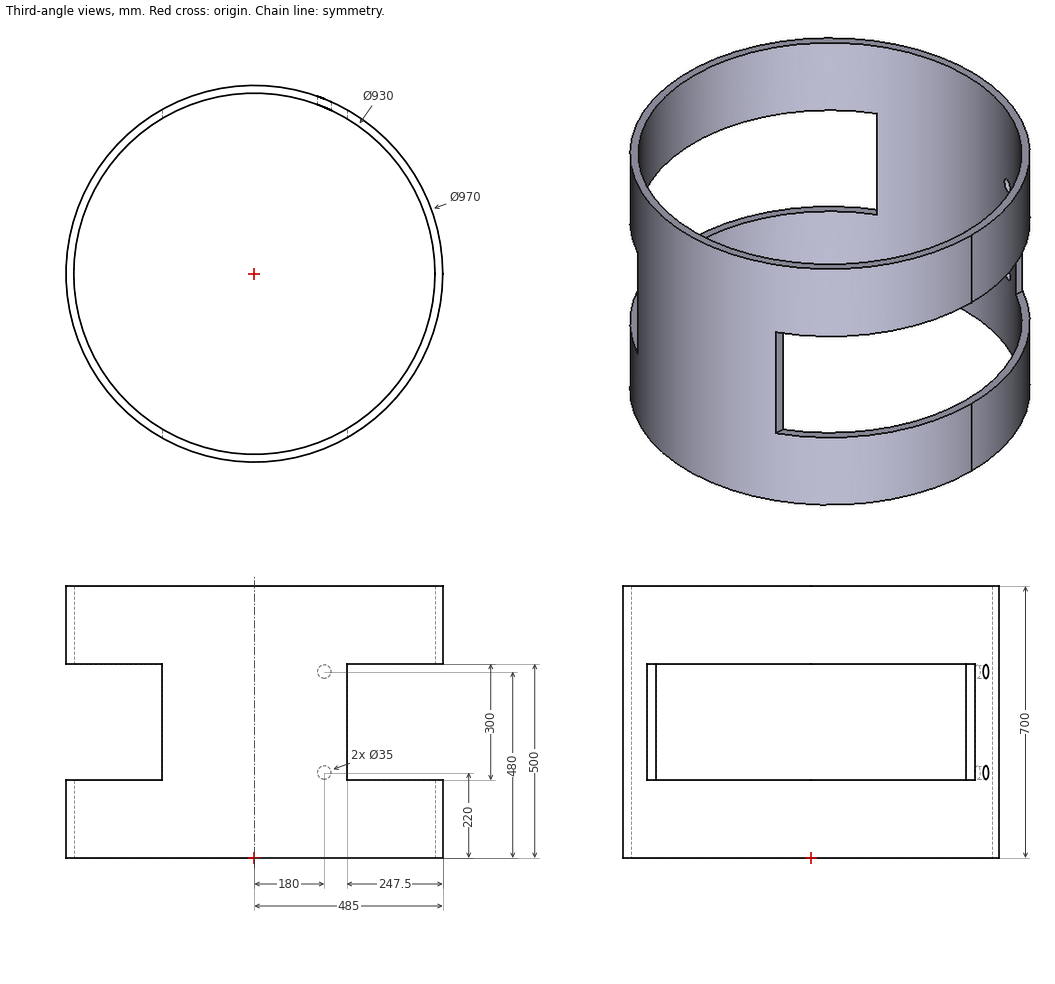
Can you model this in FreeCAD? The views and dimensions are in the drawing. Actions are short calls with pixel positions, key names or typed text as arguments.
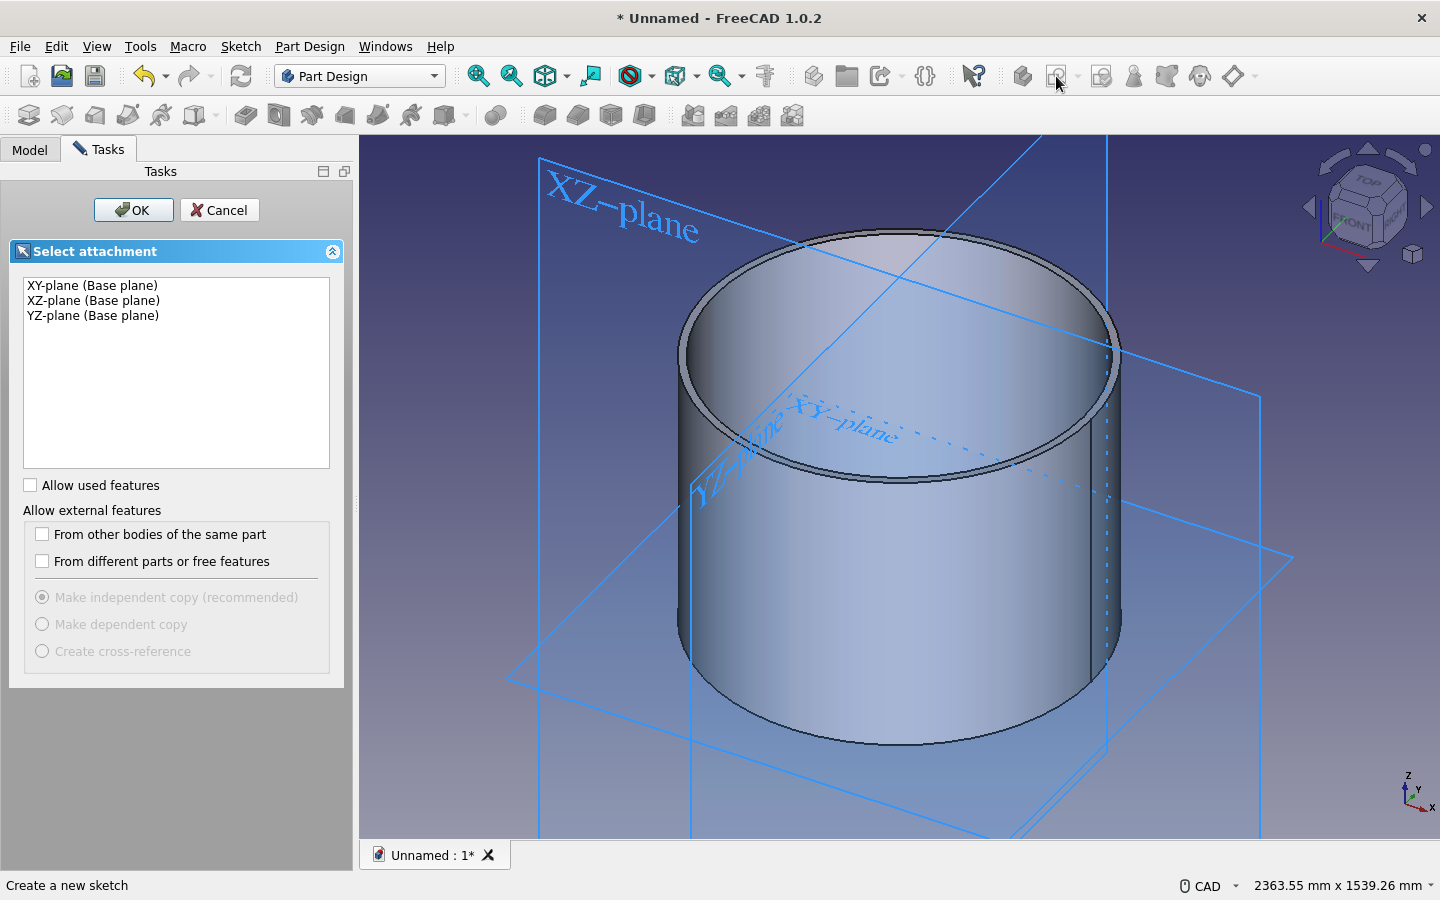
click(84, 300)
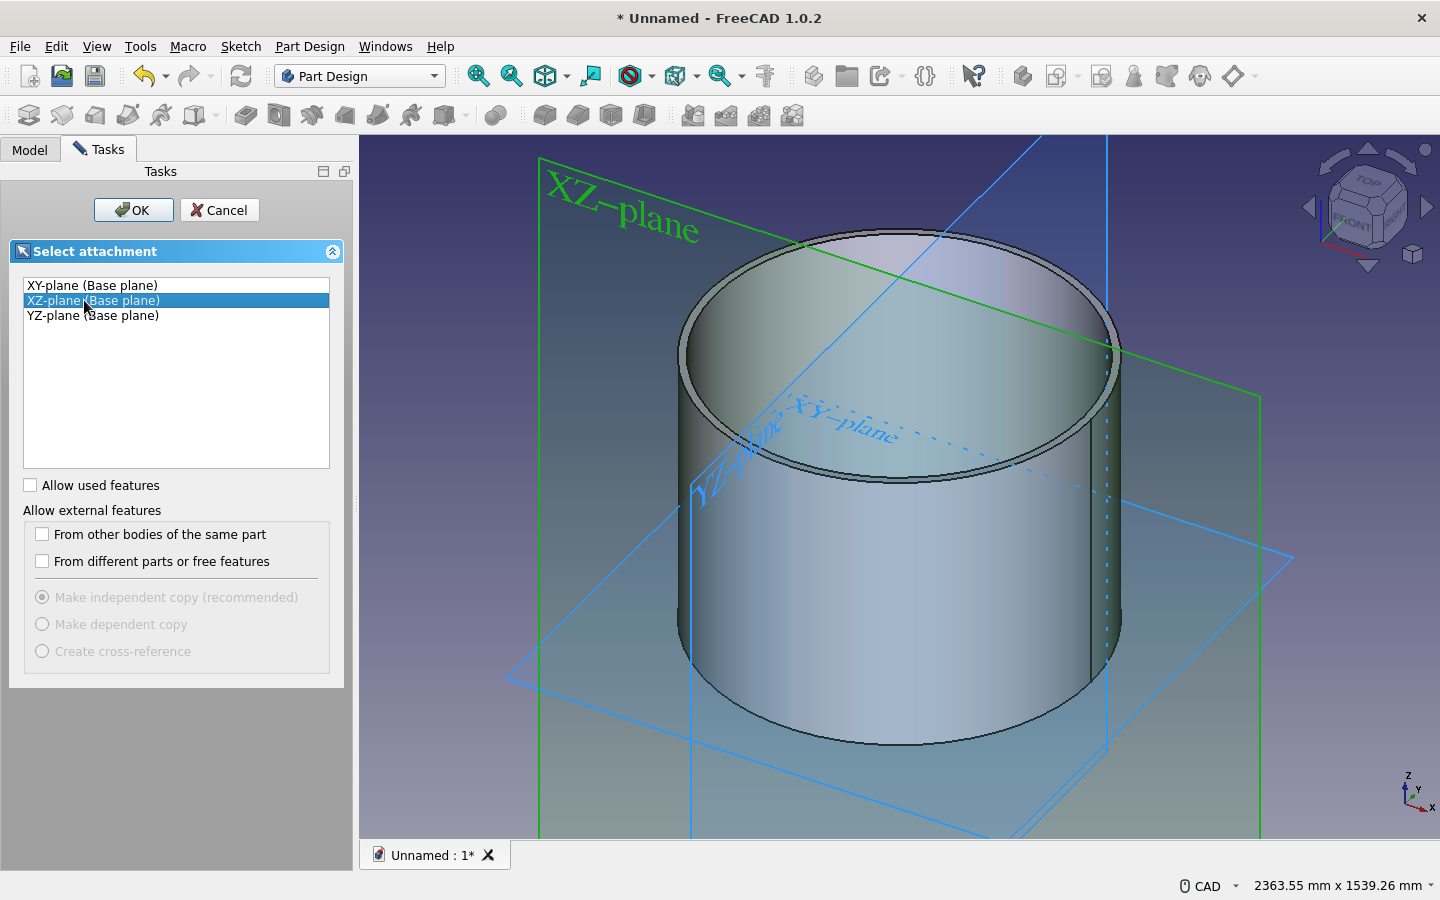
click(134, 210)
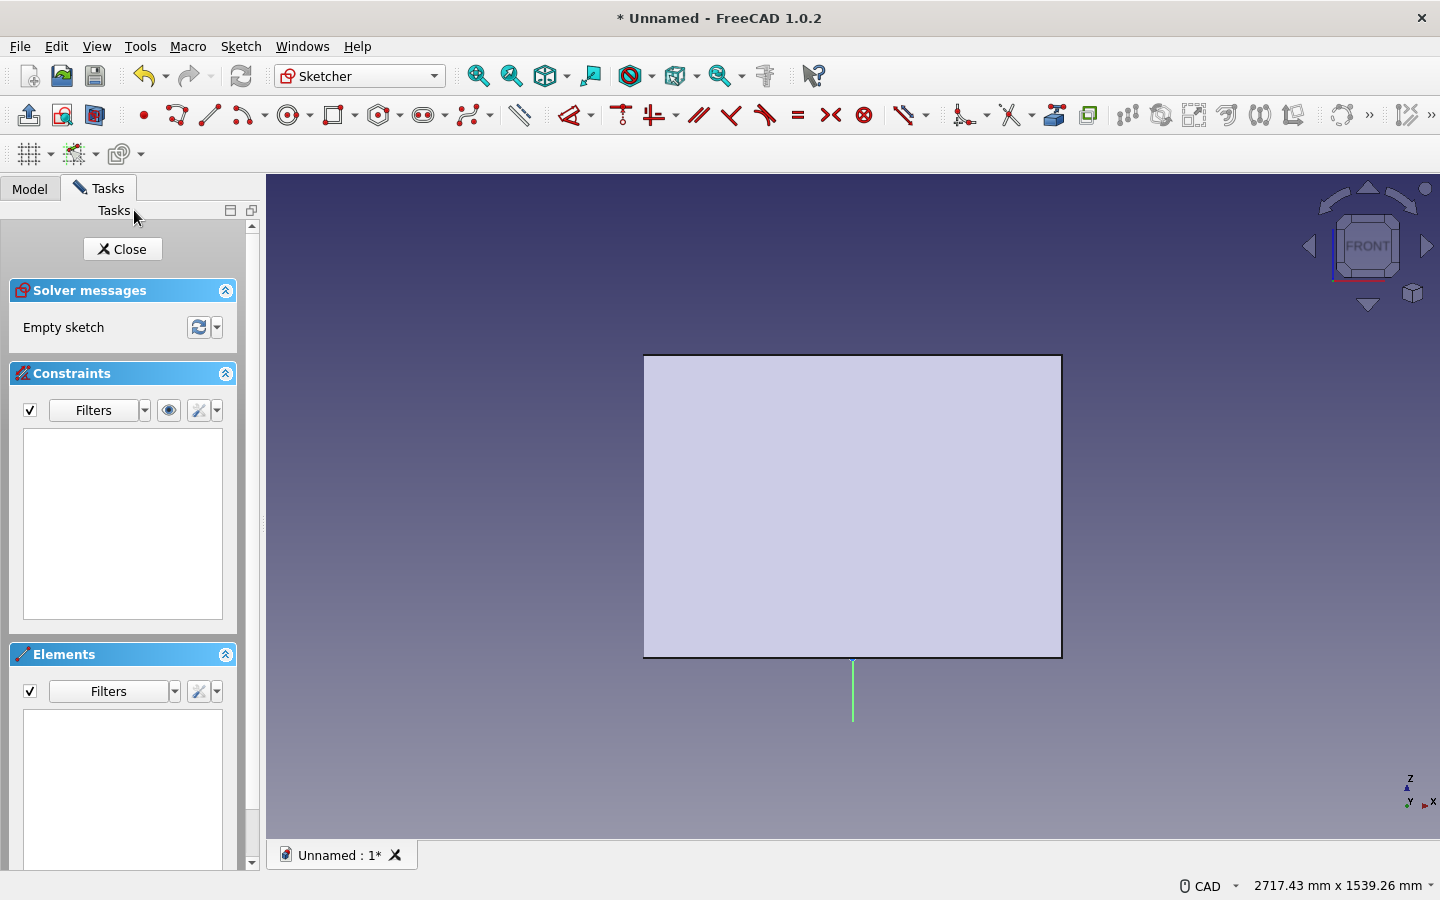
key(q)
key(s)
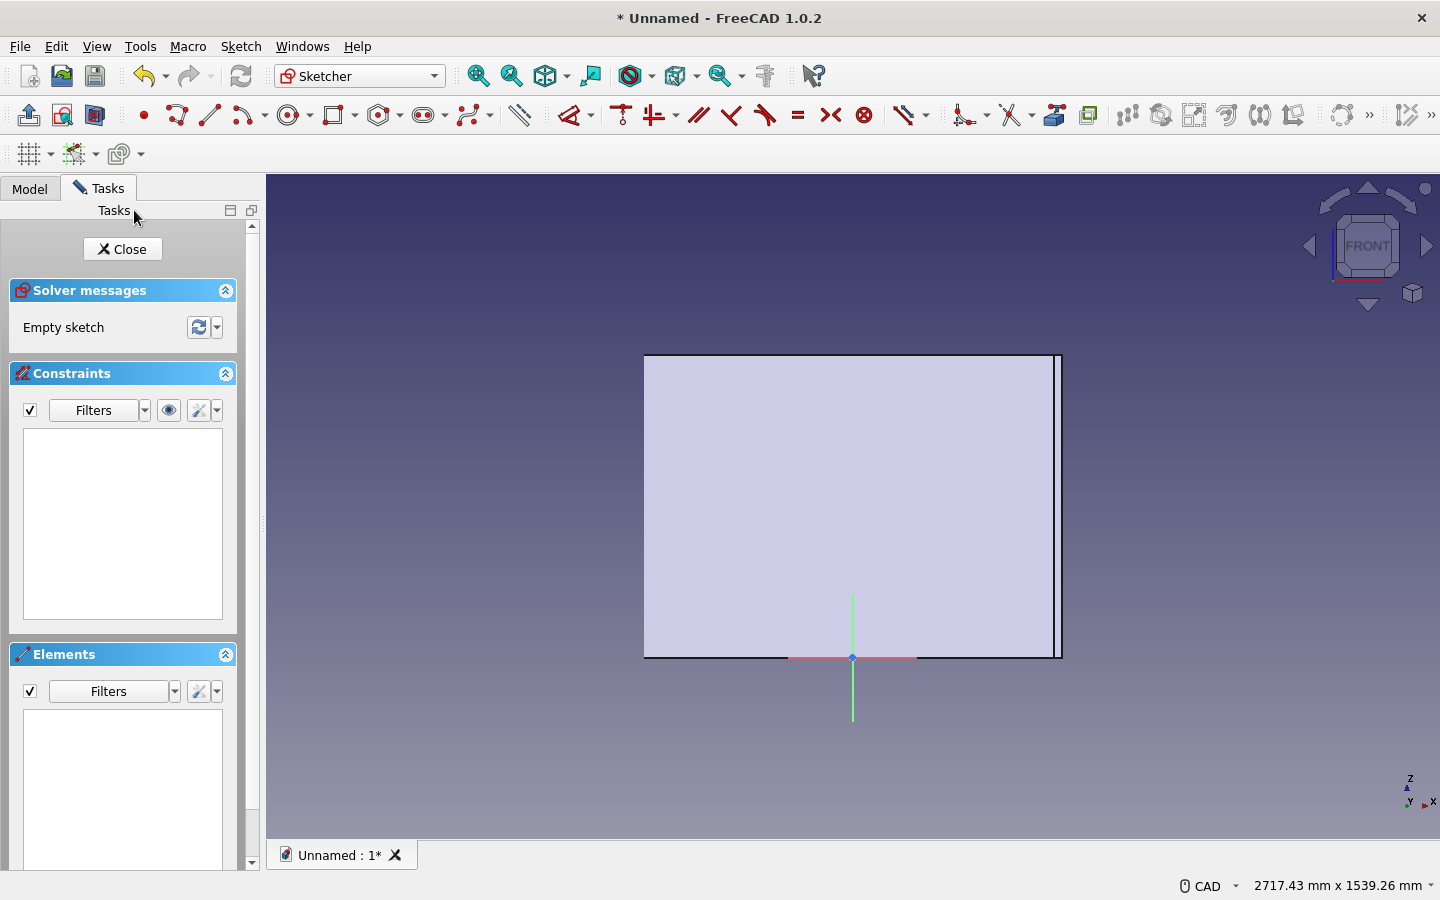
scroll(936, 602, up, 3)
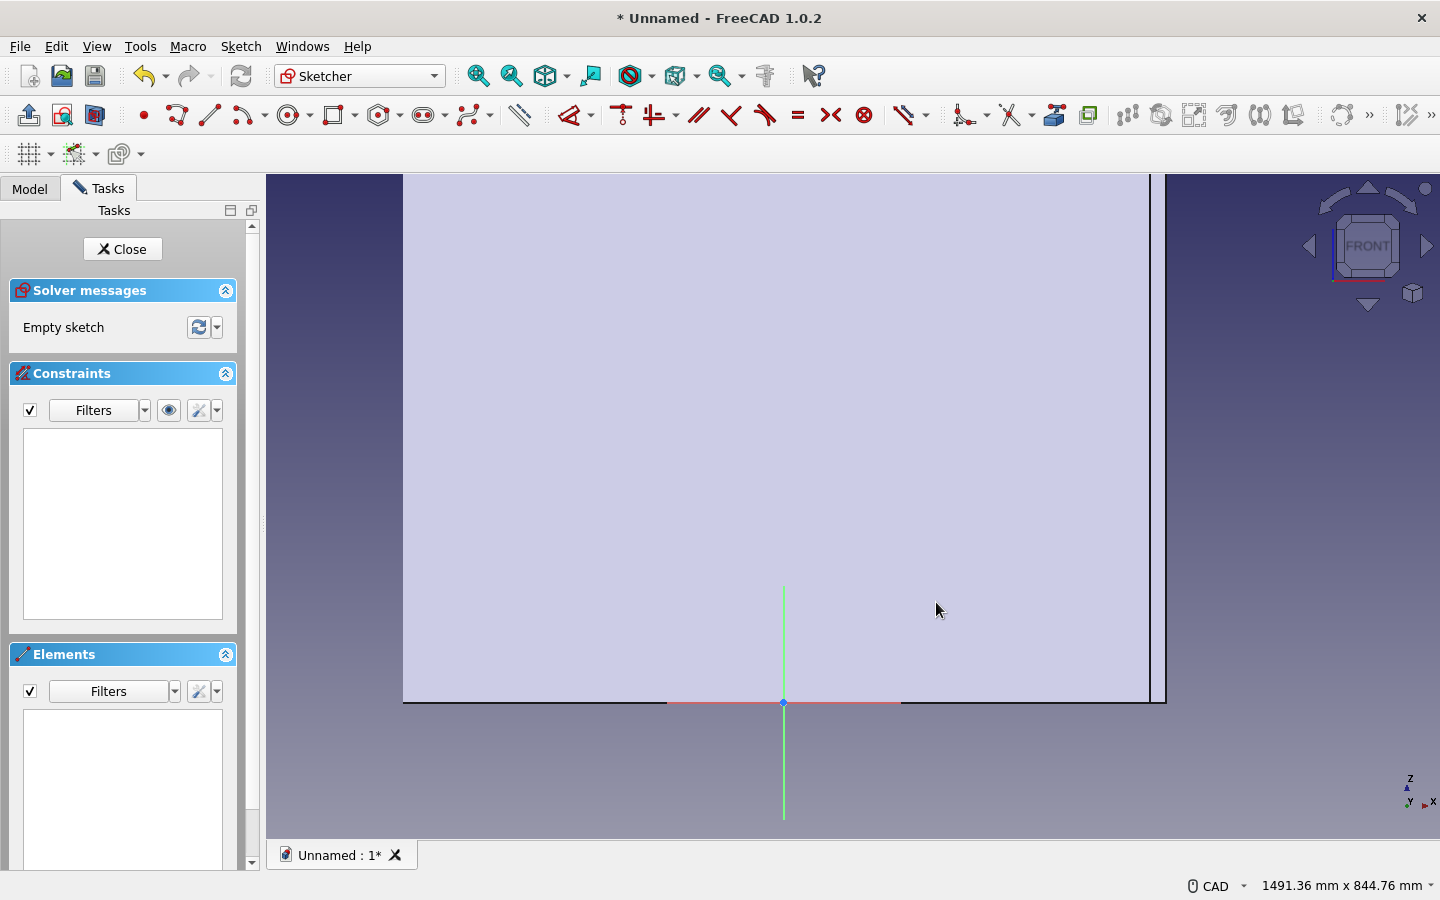
key(g)
key(r)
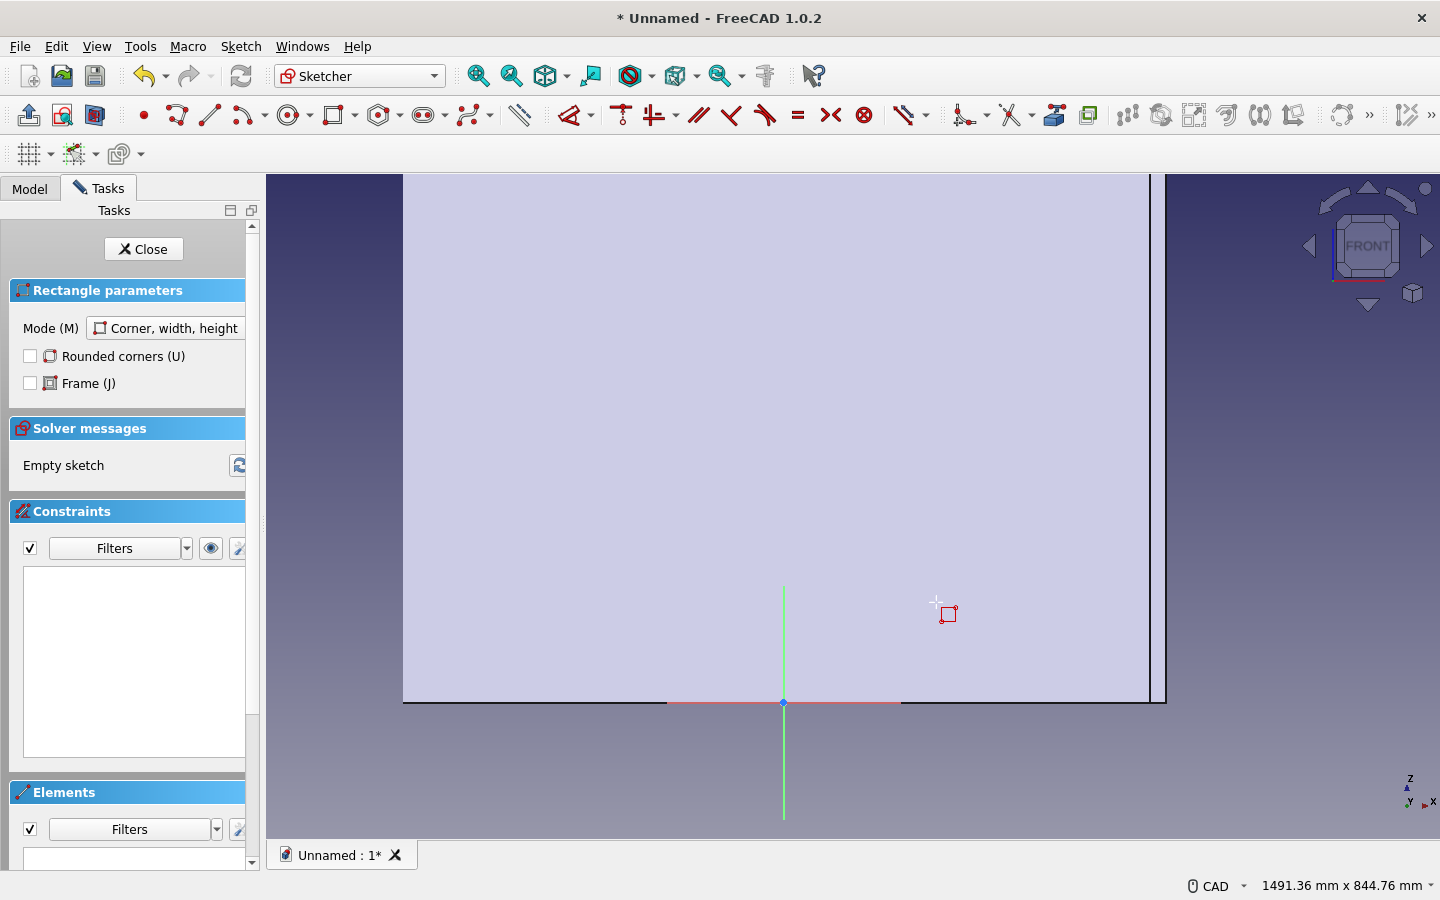
click(971, 309)
click(1166, 546)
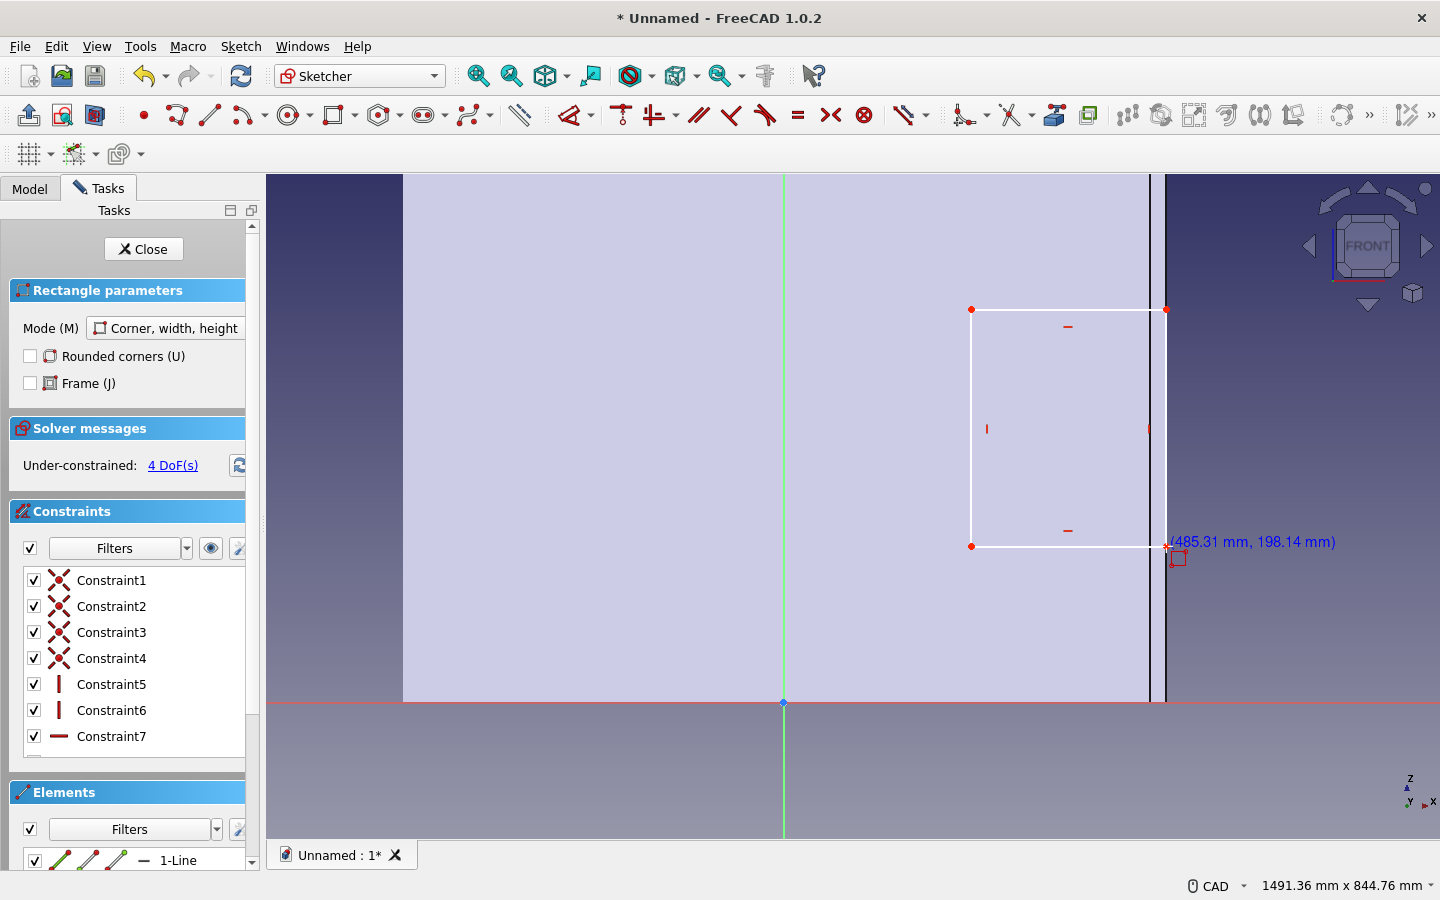
click(402, 309)
click(597, 546)
key(Escape)